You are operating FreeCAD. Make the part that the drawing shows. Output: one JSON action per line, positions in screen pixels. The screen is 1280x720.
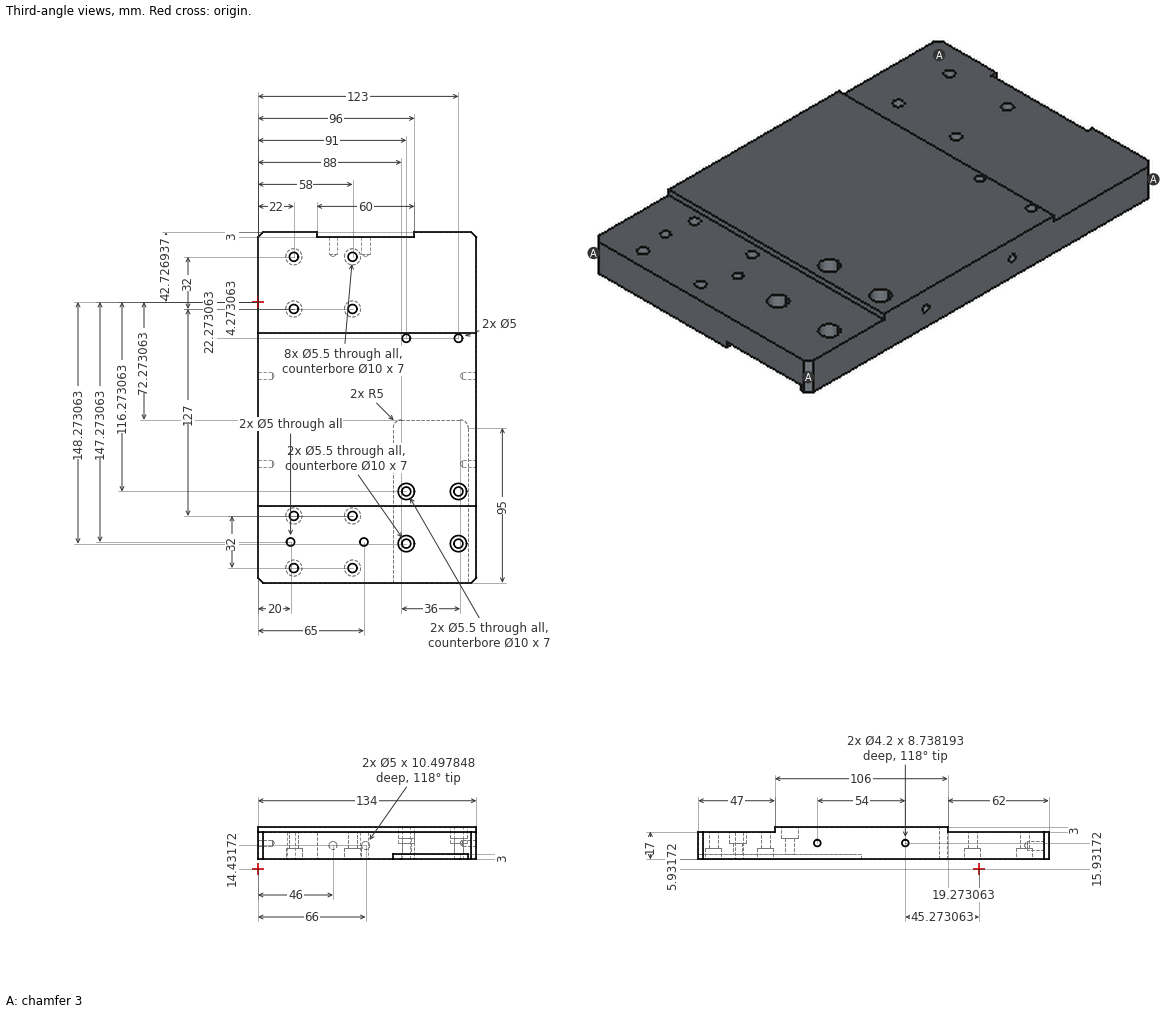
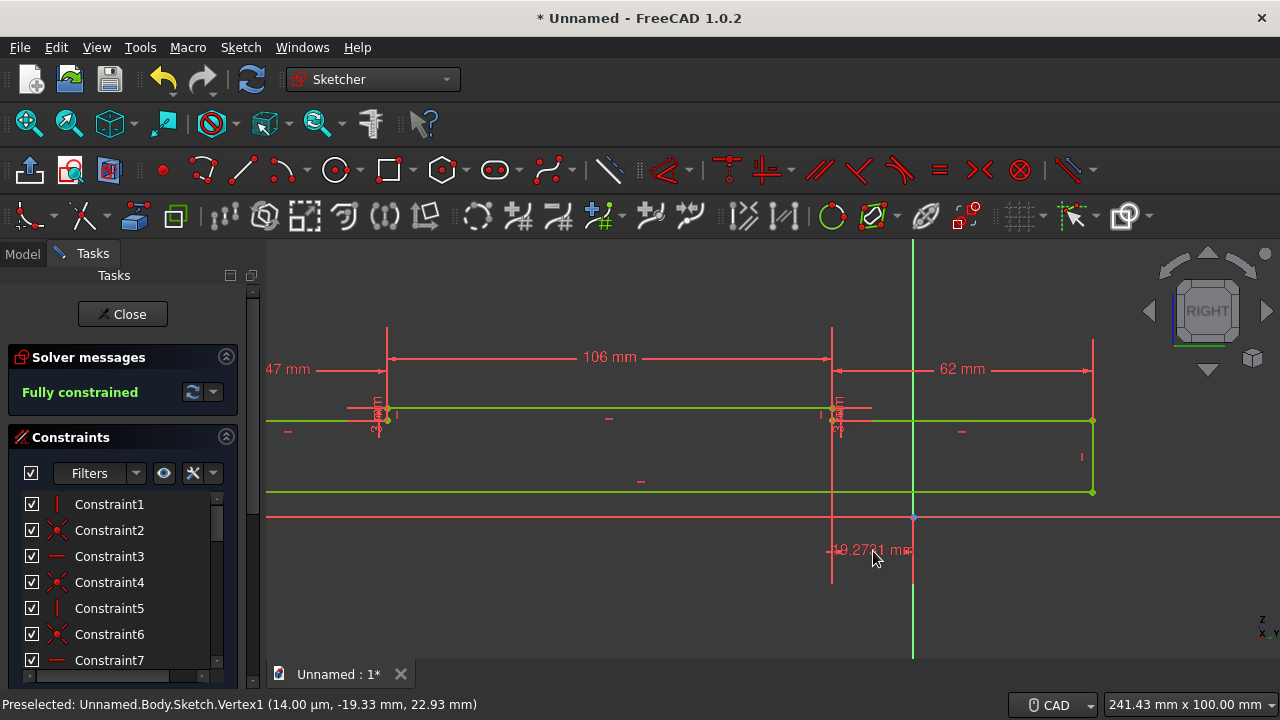
{"action": "left_click", "coordinate": [123, 314]}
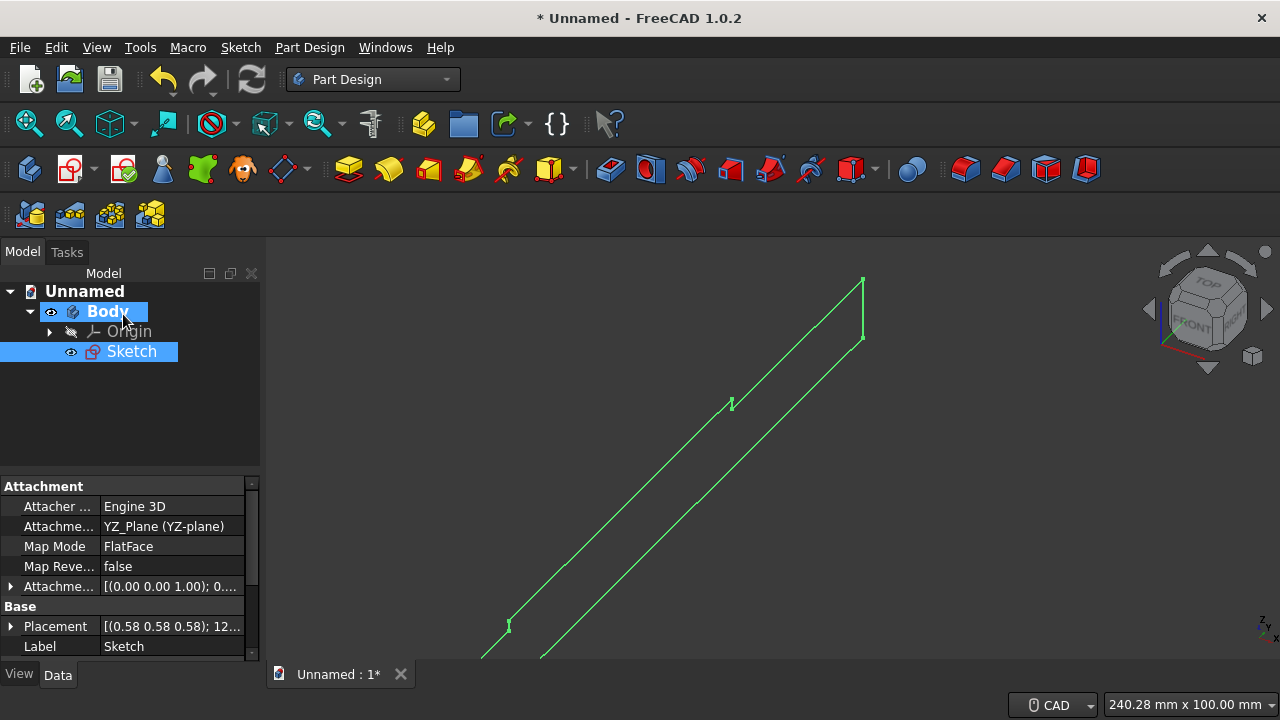
{"action": "left_click", "coordinate": [350, 170]}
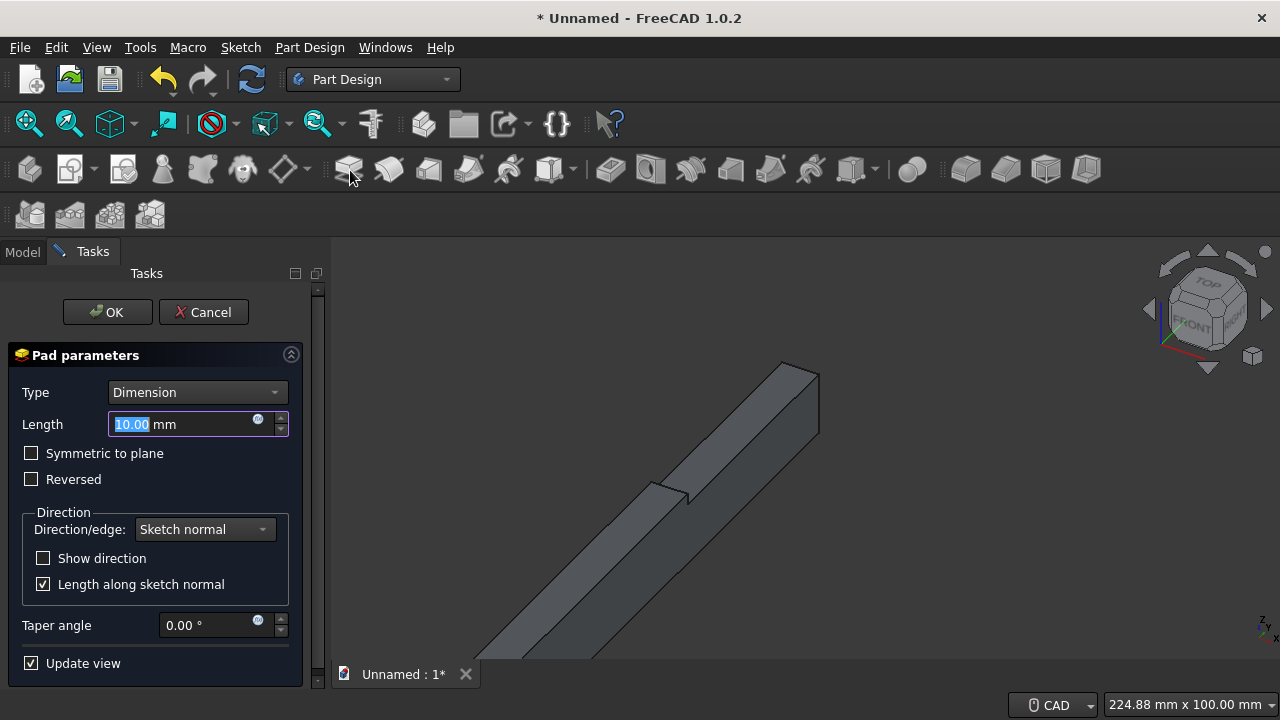
{"action": "type", "text": "134"}
{"action": "key", "text": "Tab"}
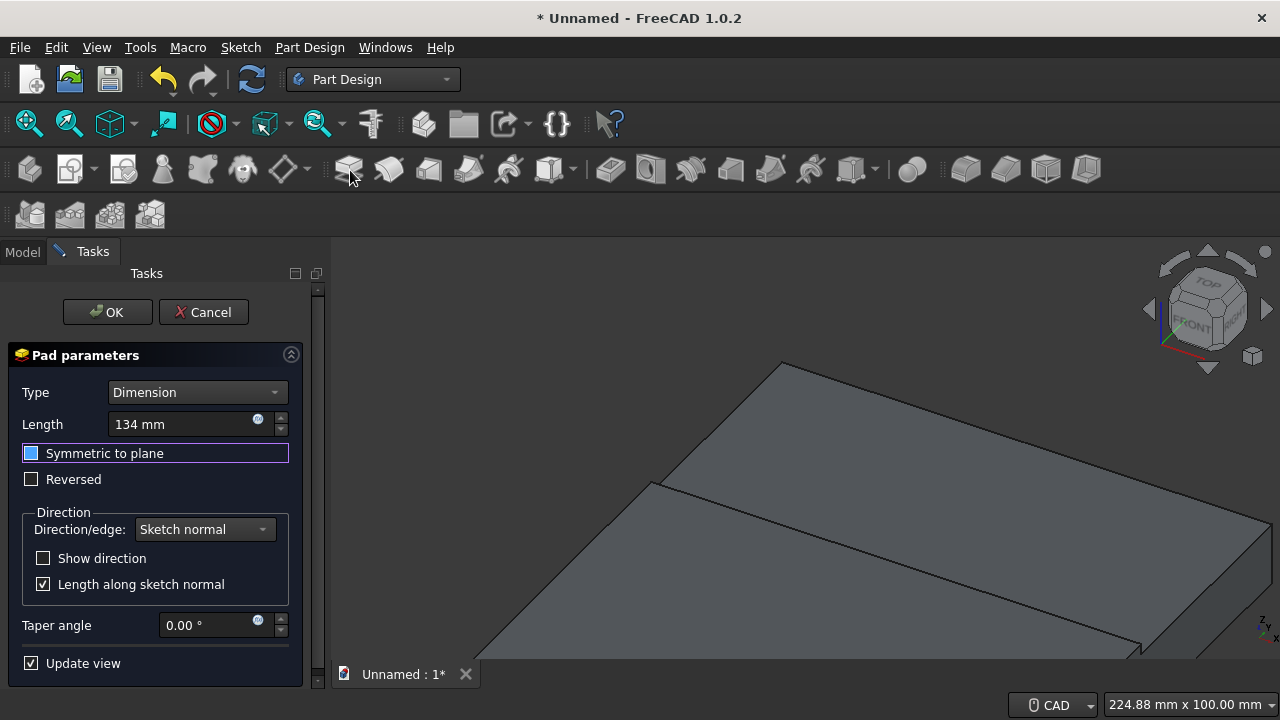
{"action": "left_click", "coordinate": [108, 312]}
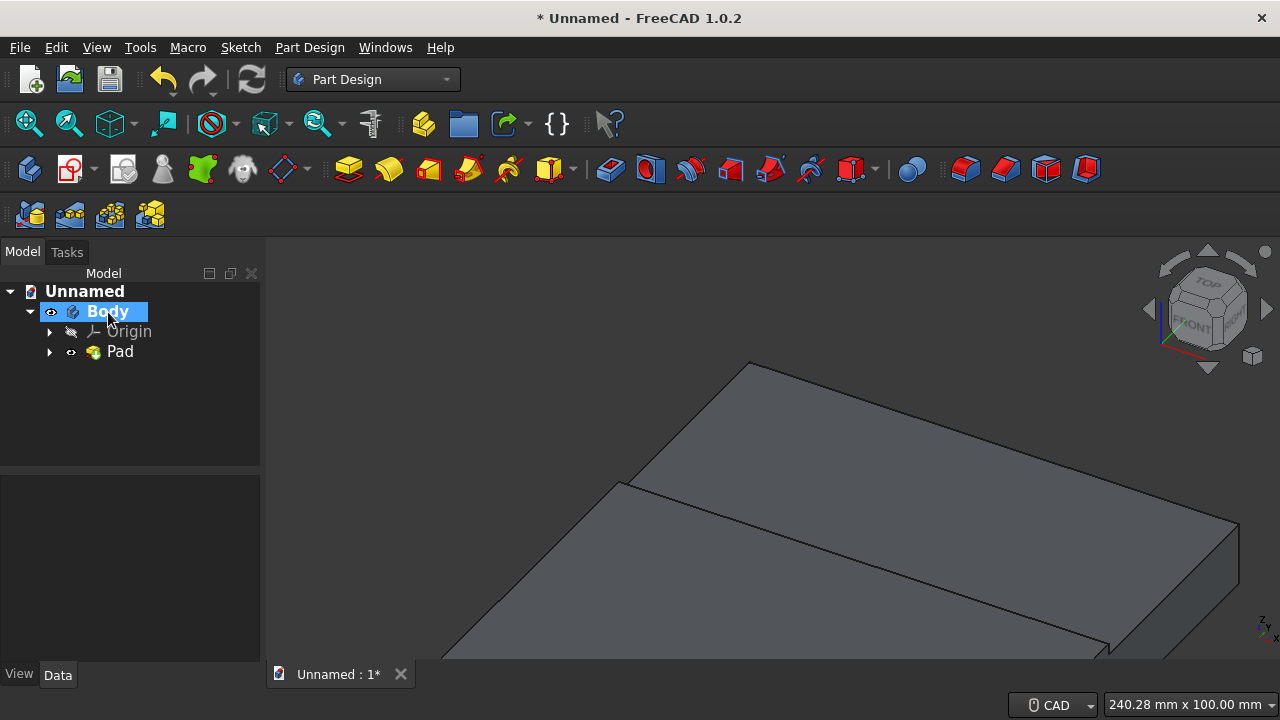
{"action": "left_click", "coordinate": [30, 124]}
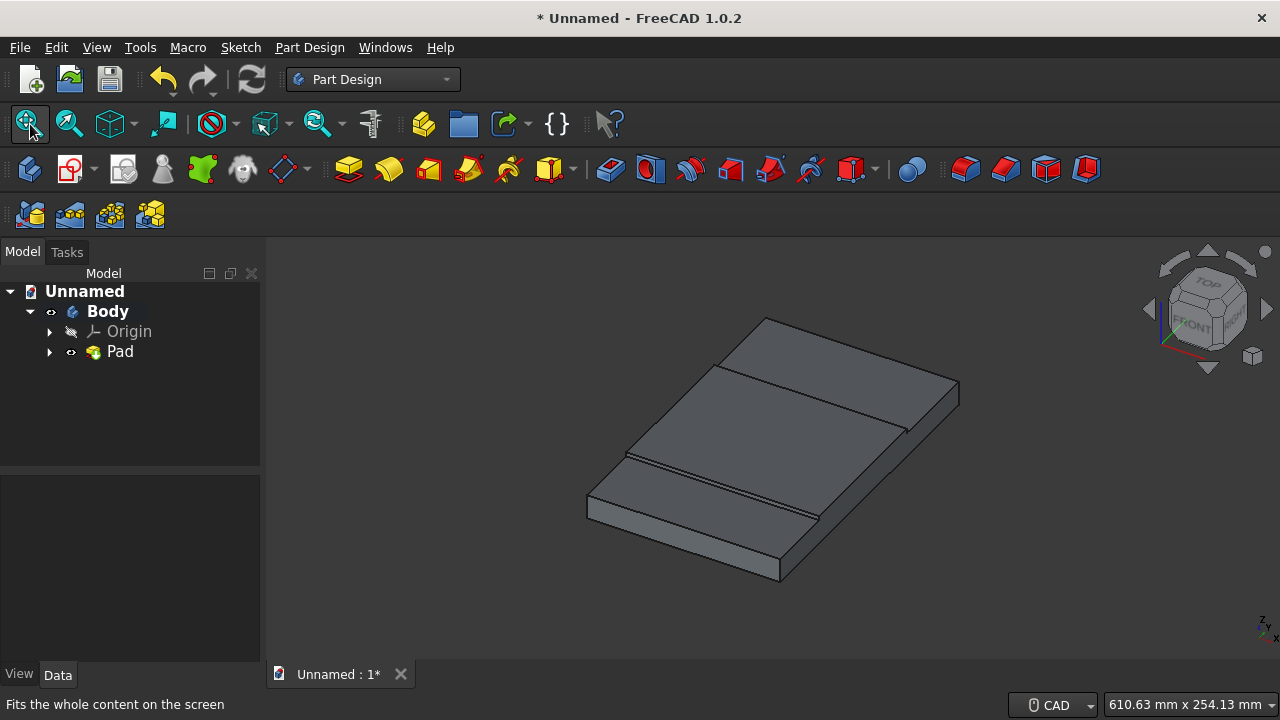
{"action": "left_click", "coordinate": [864, 383]}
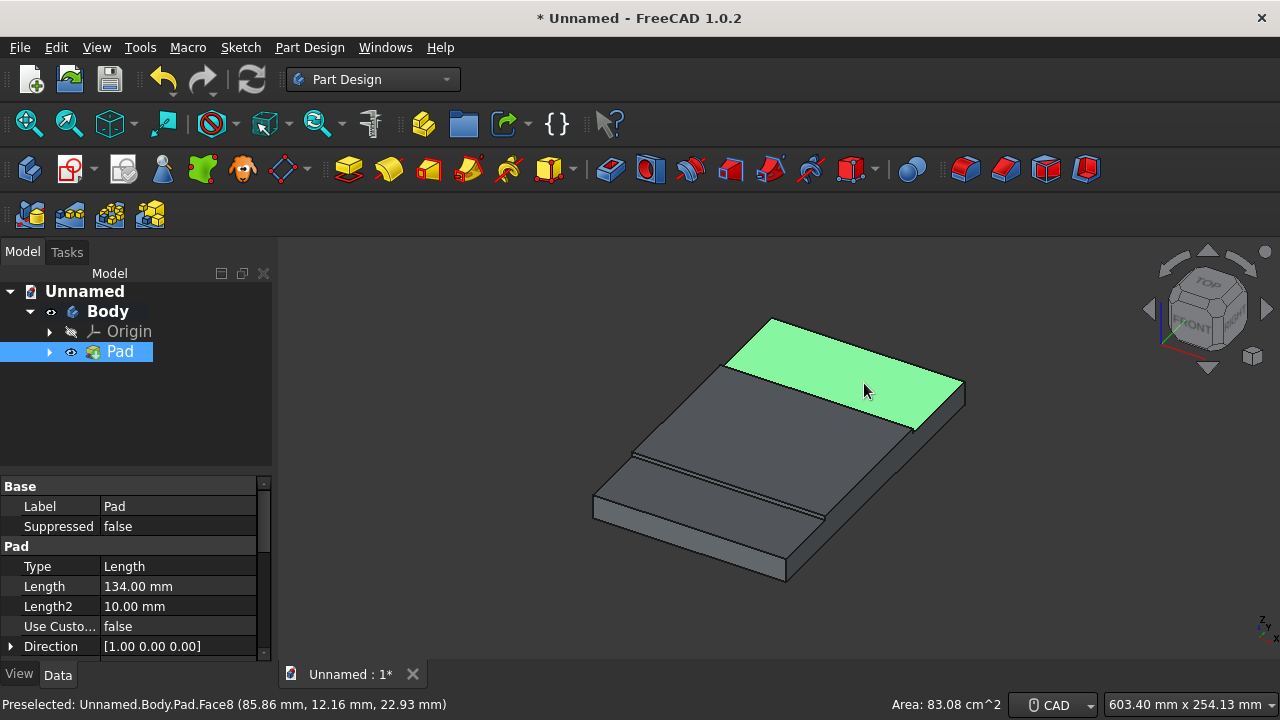
{"action": "left_click", "coordinate": [70, 170]}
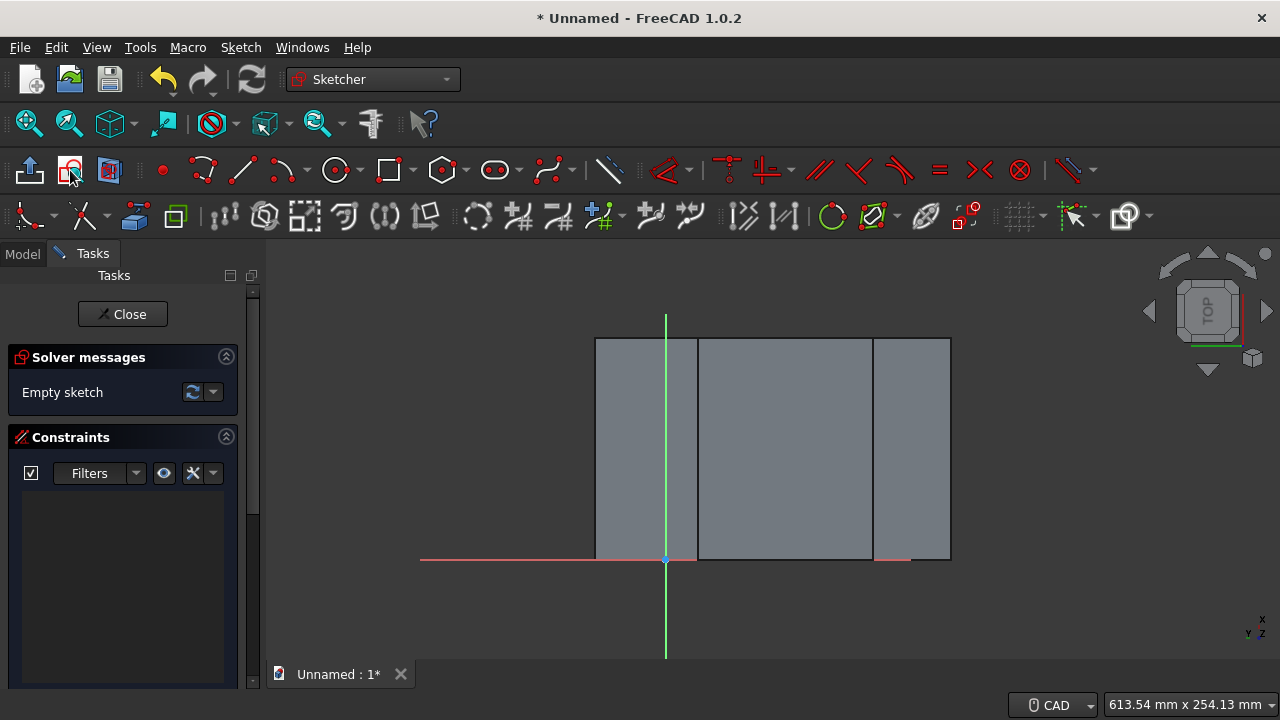
{"action": "scroll", "coordinate": [480, 544], "scroll_direction": "up", "scroll_amount": 2}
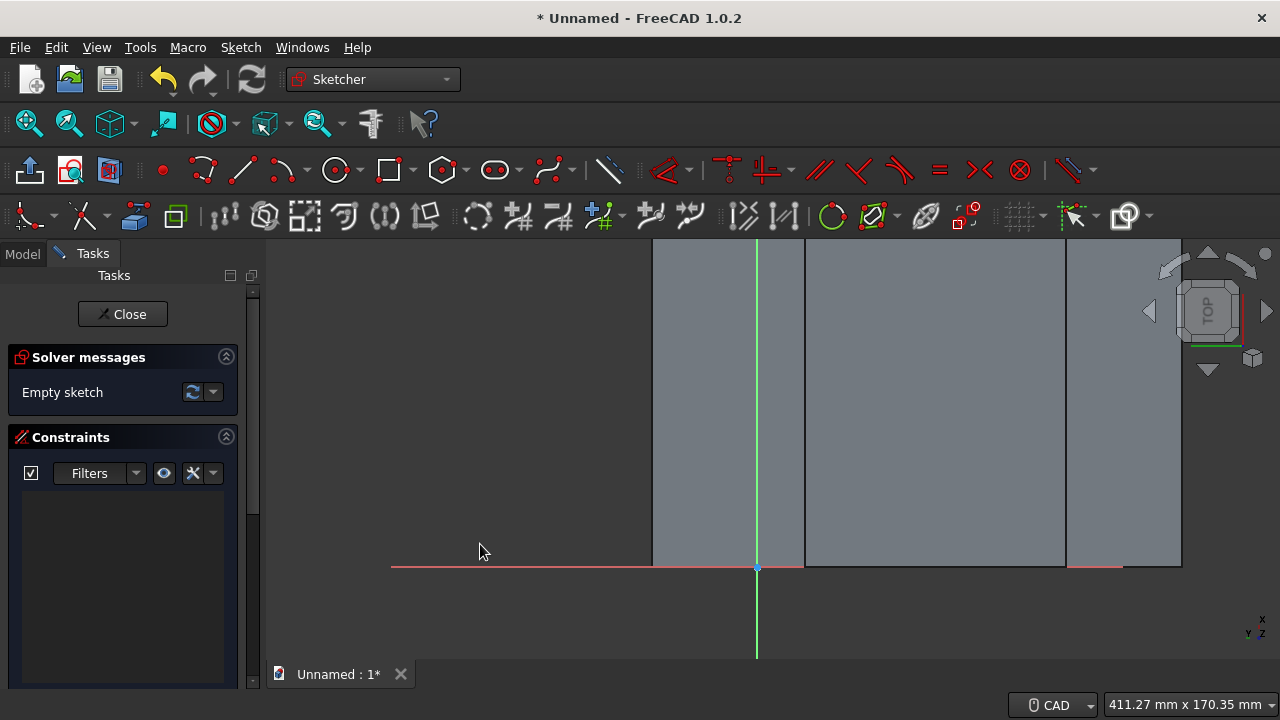
{"action": "left_click", "coordinate": [390, 170]}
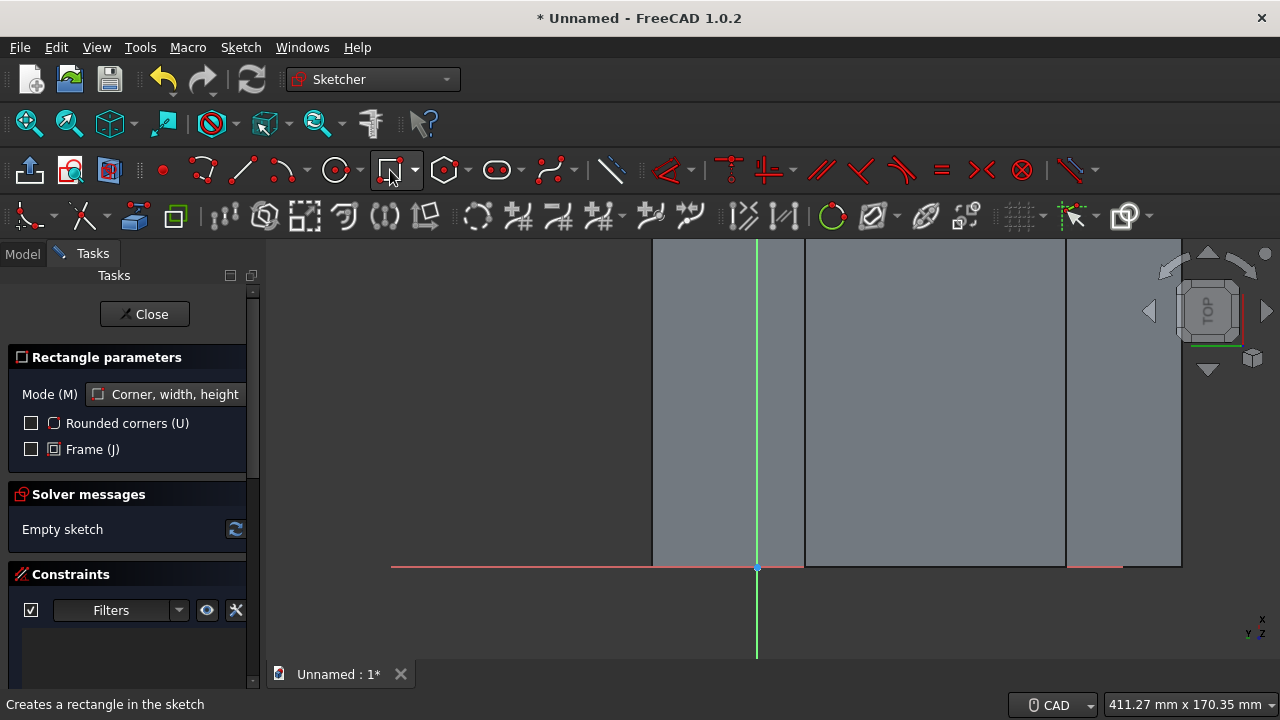
{"action": "scroll", "coordinate": [652, 330], "scroll_direction": "up", "scroll_amount": 4}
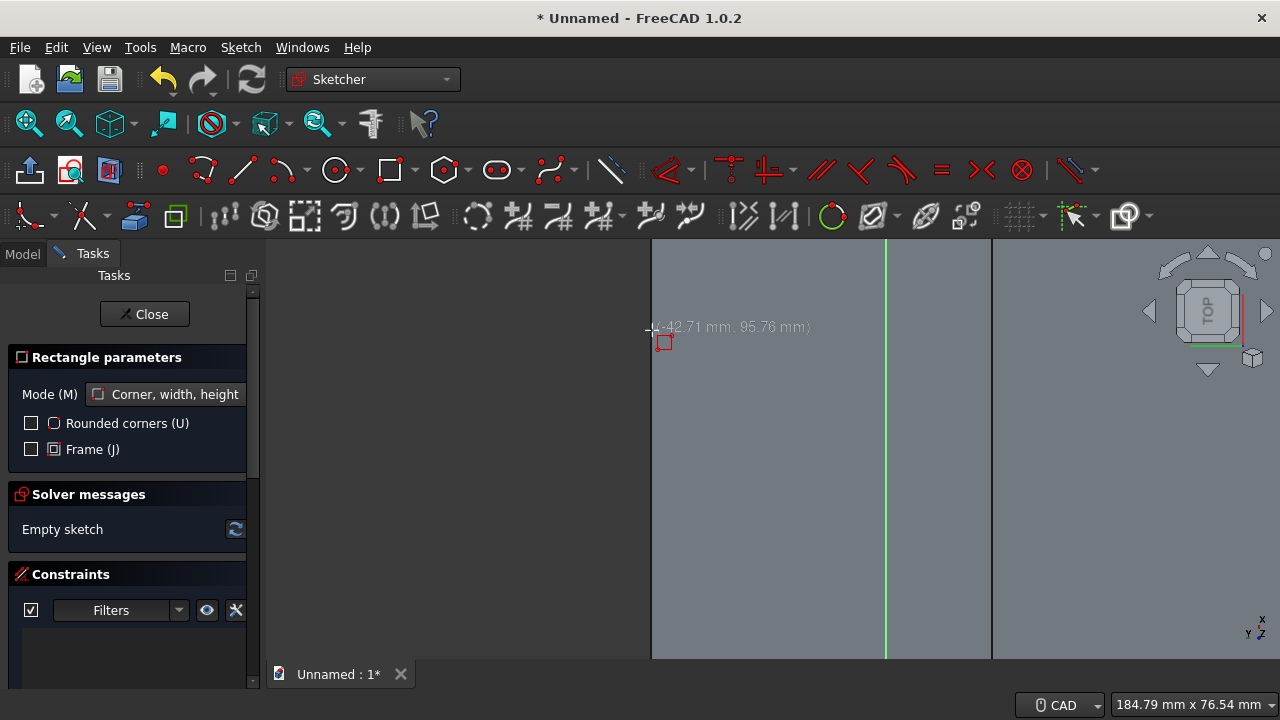
{"action": "left_click", "coordinate": [651, 331]}